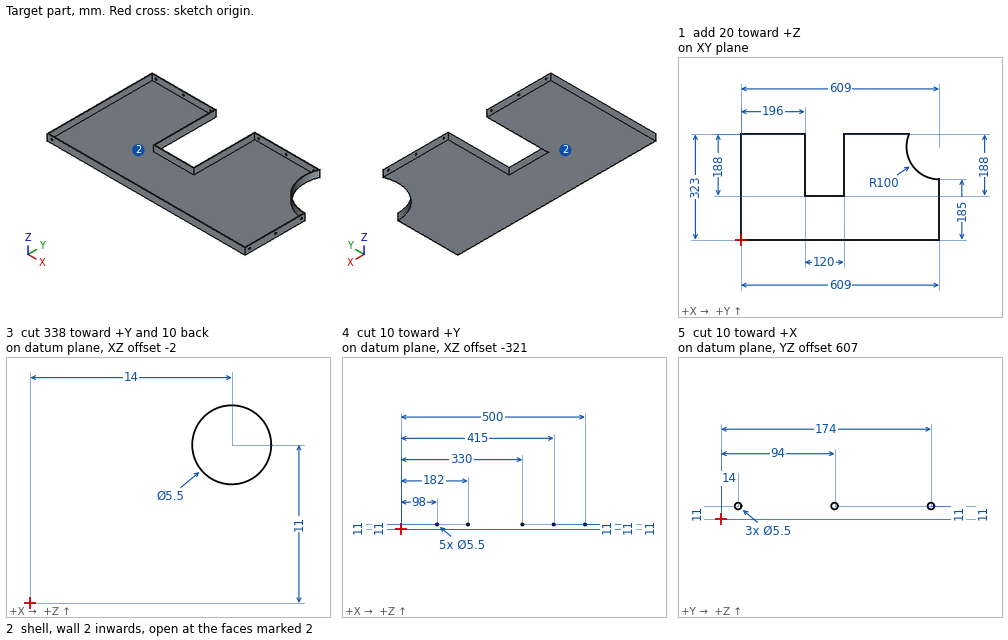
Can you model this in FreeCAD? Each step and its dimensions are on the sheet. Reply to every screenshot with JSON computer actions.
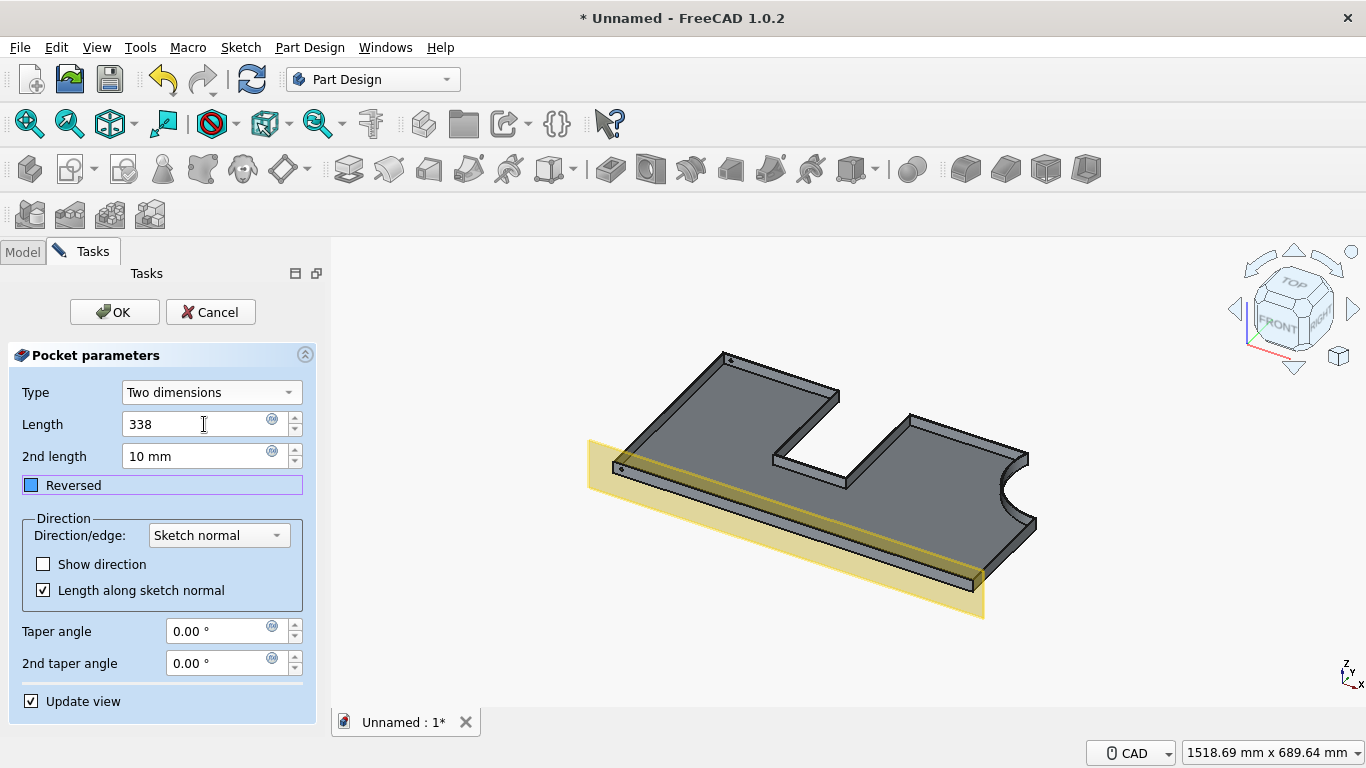
{"action": "left_click", "coordinate": [115, 312]}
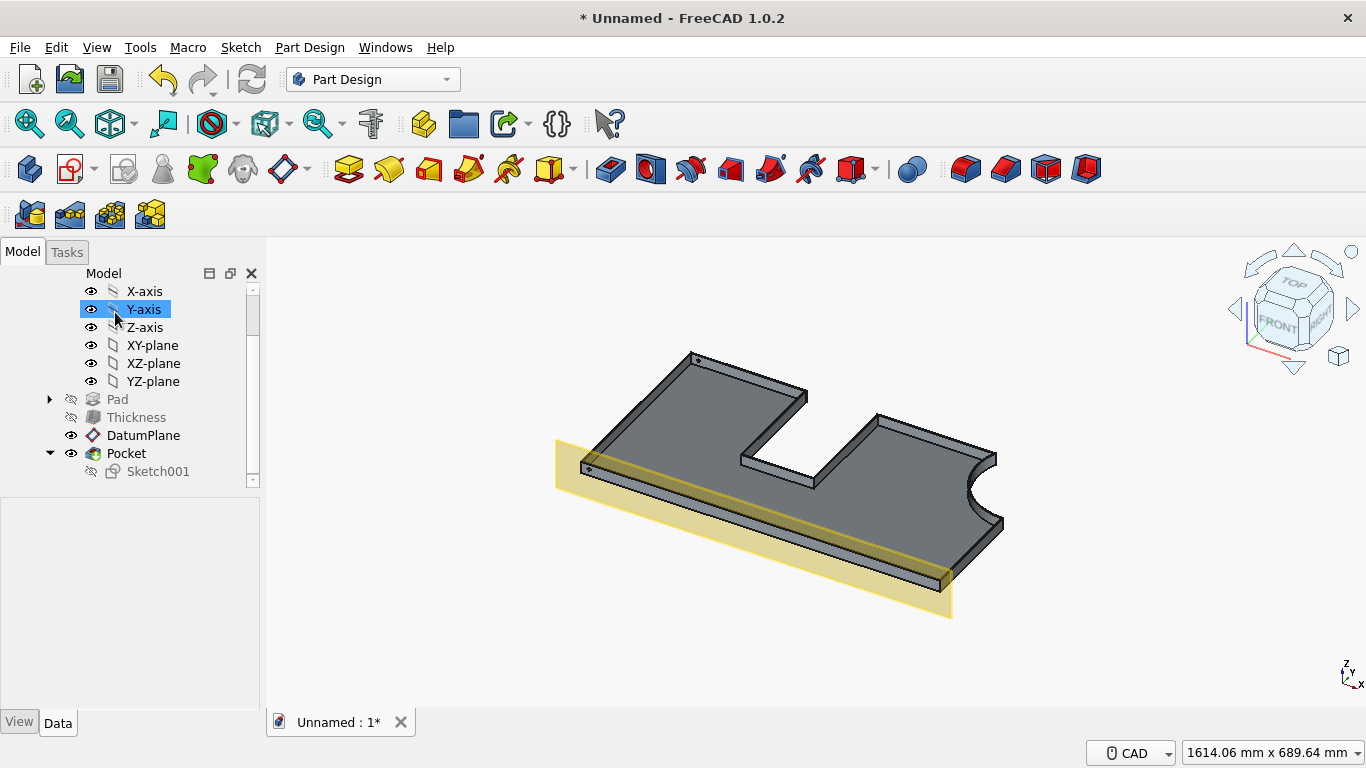
{"action": "left_click", "coordinate": [116, 435]}
{"action": "key", "text": "space"}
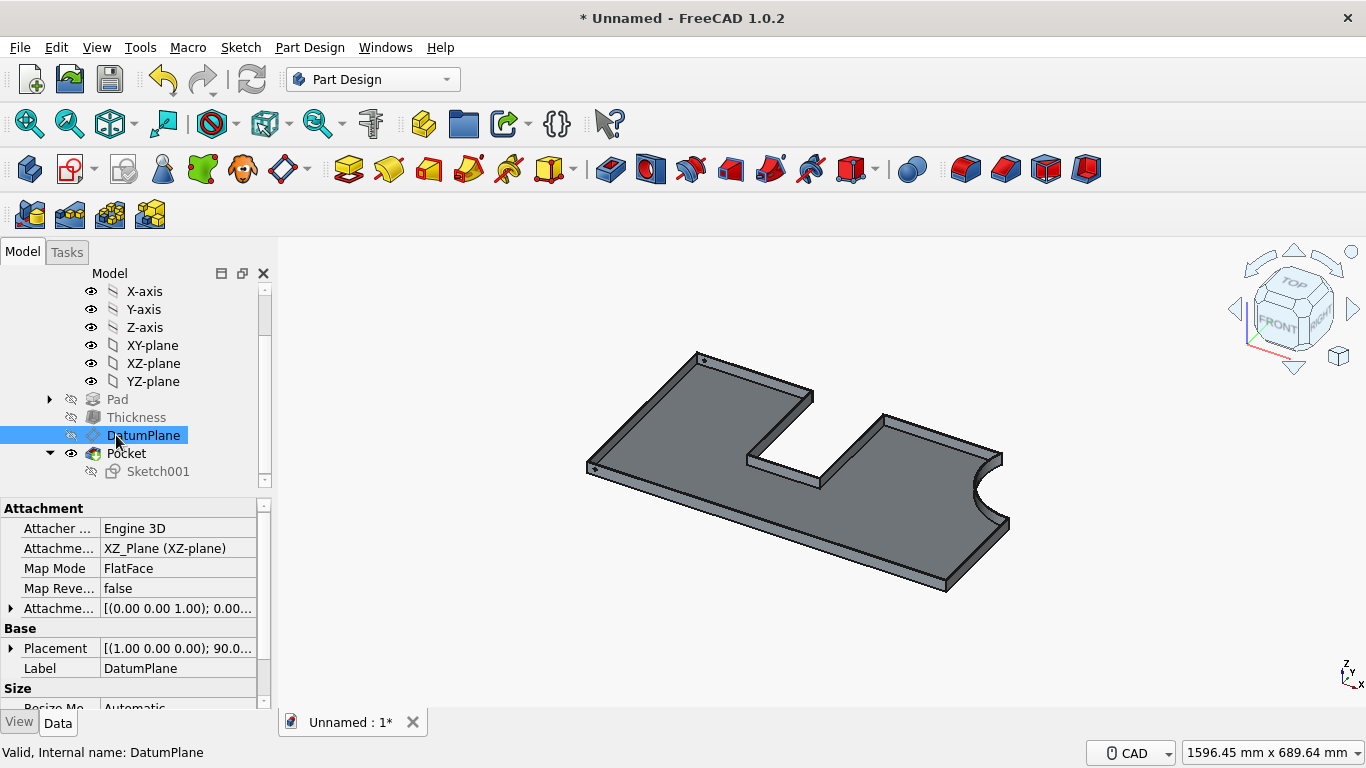
{"action": "scroll", "coordinate": [160, 377], "scroll_direction": "down", "scroll_amount": 3}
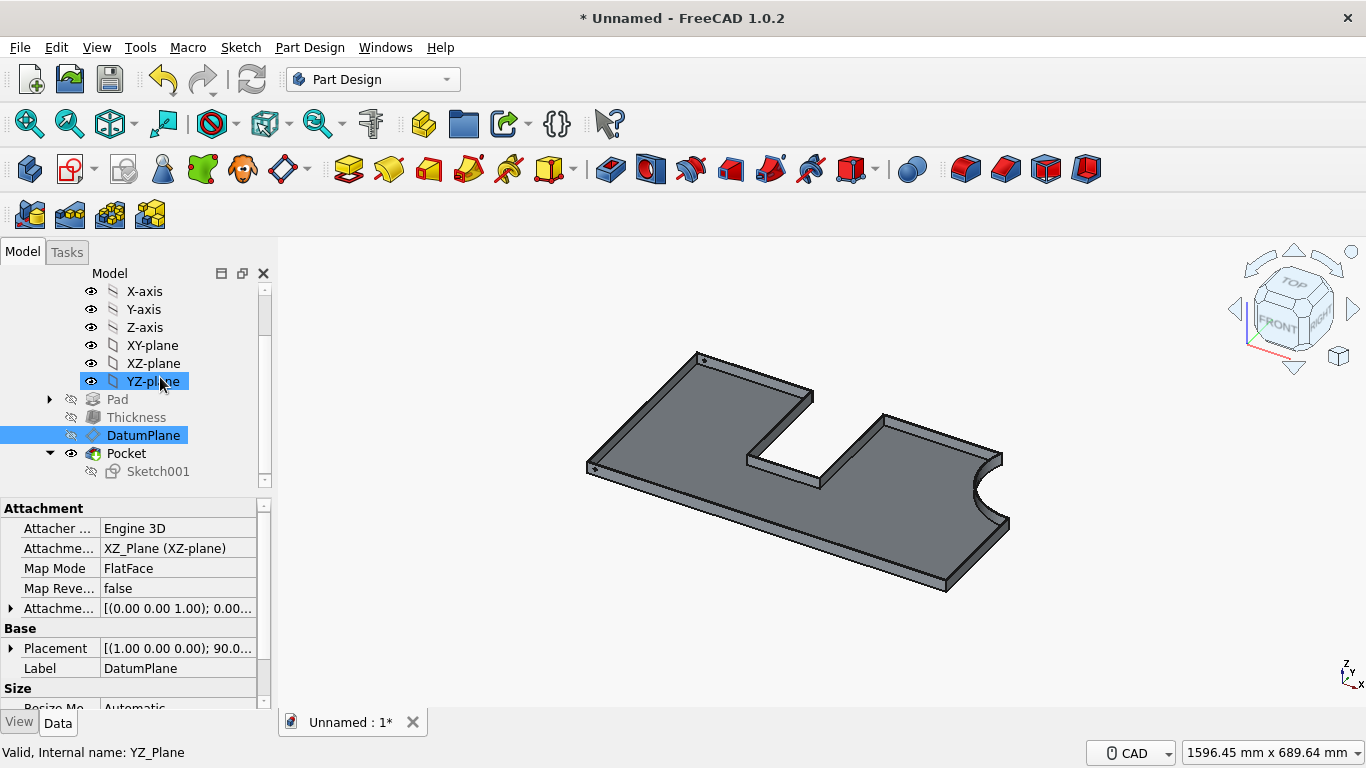
{"action": "scroll", "coordinate": [160, 377], "scroll_direction": "up", "scroll_amount": 15}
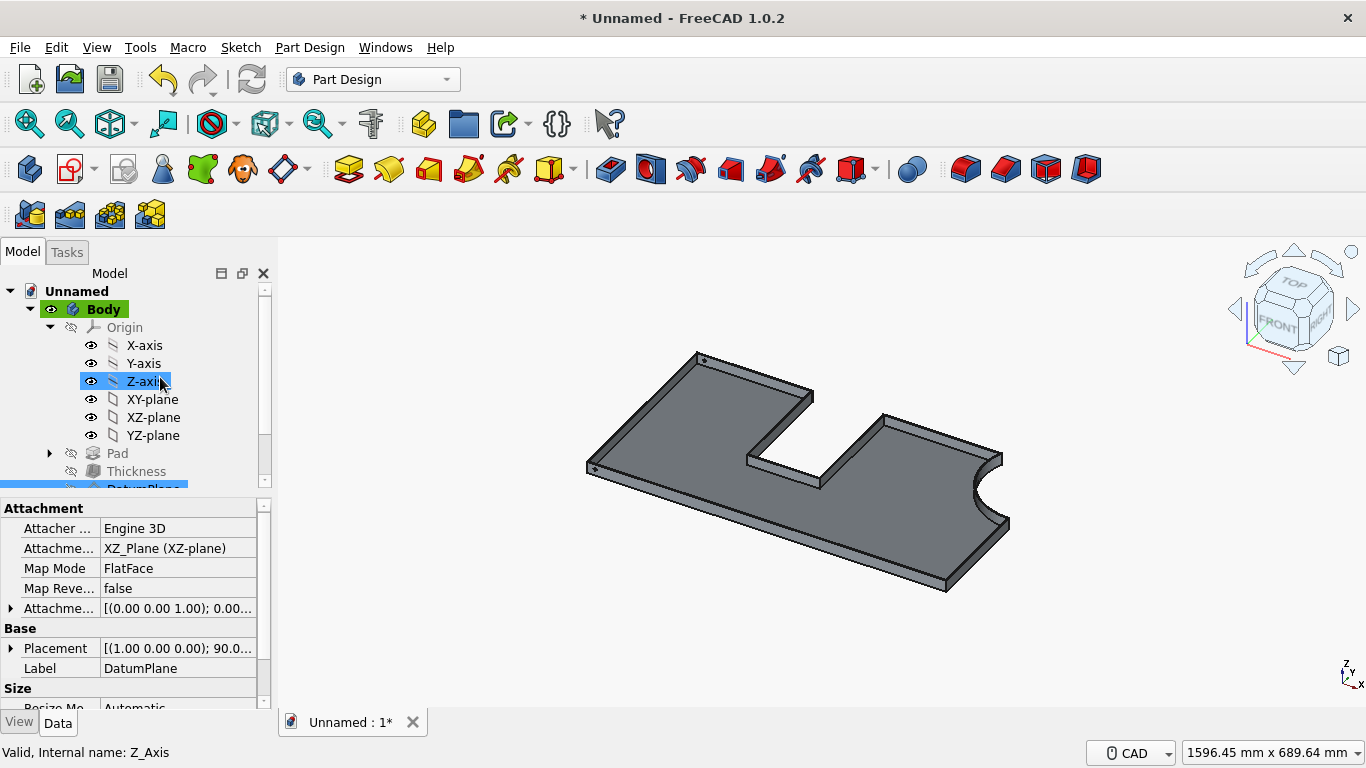
{"action": "left_click", "coordinate": [136, 417]}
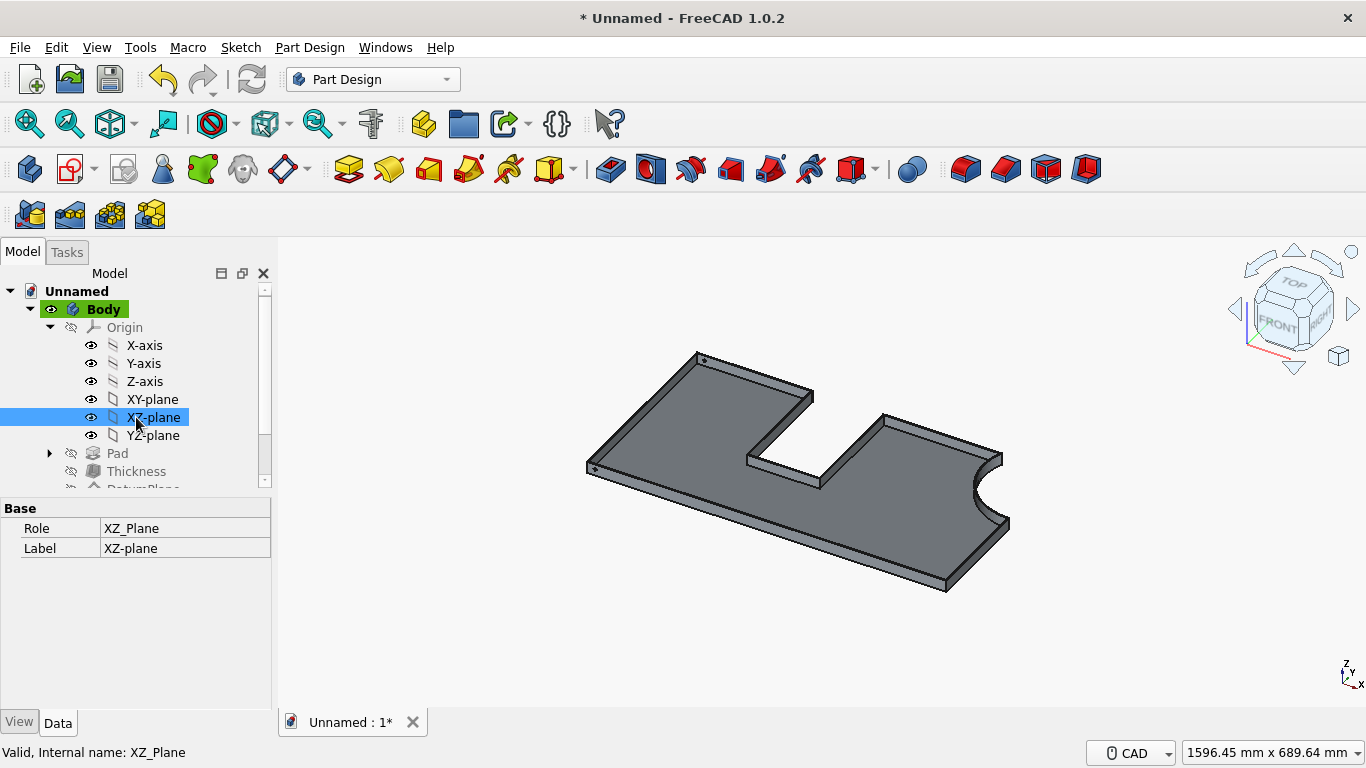
{"action": "left_click", "coordinate": [284, 170]}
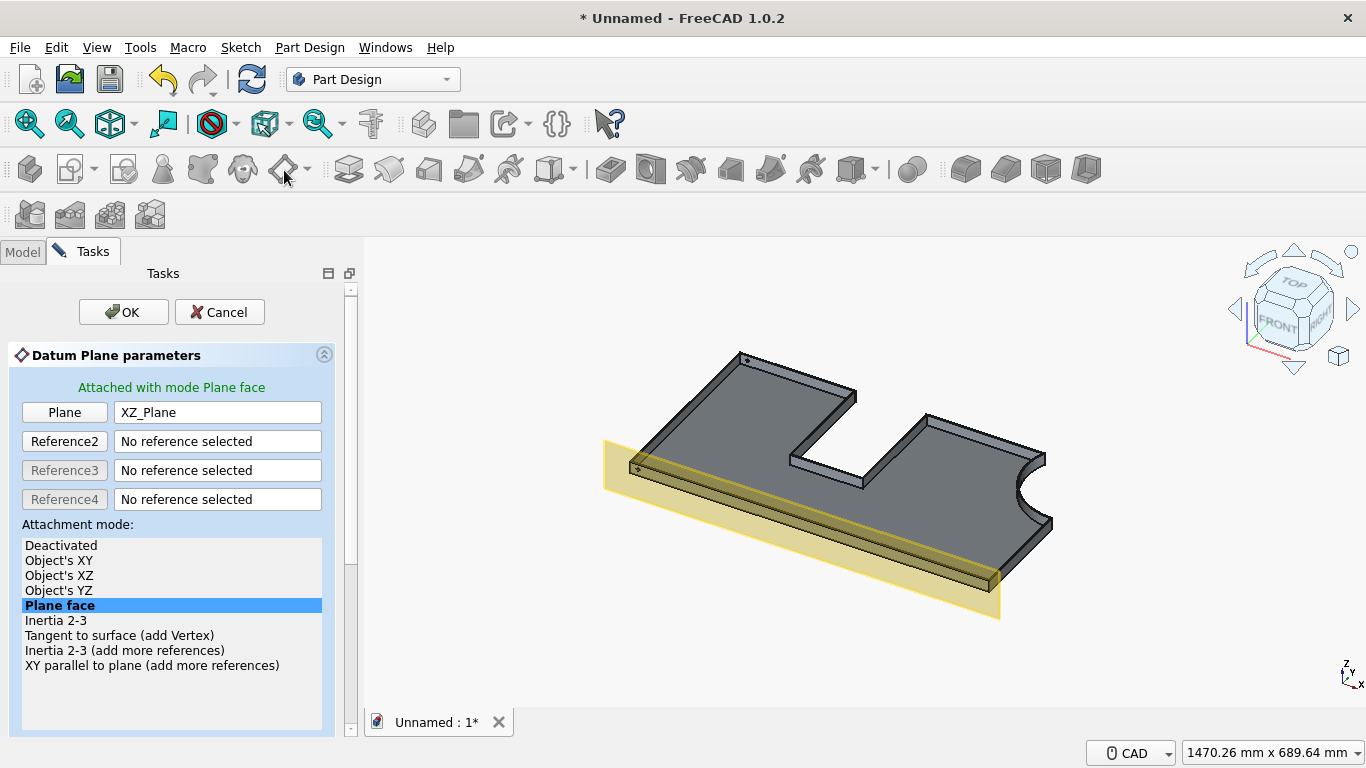
{"action": "scroll", "coordinate": [351, 510], "scroll_direction": "down", "scroll_amount": 3}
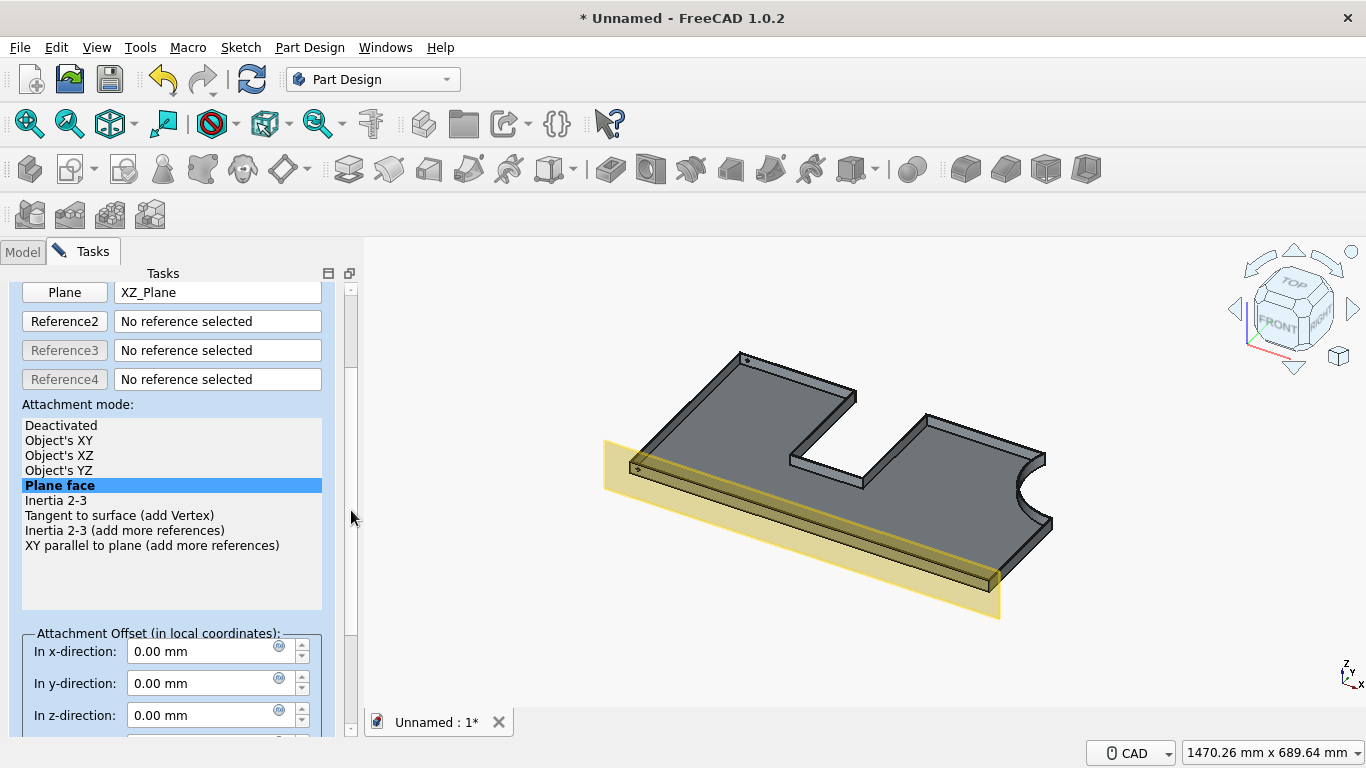
{"action": "triple_click", "coordinate": [210, 655]}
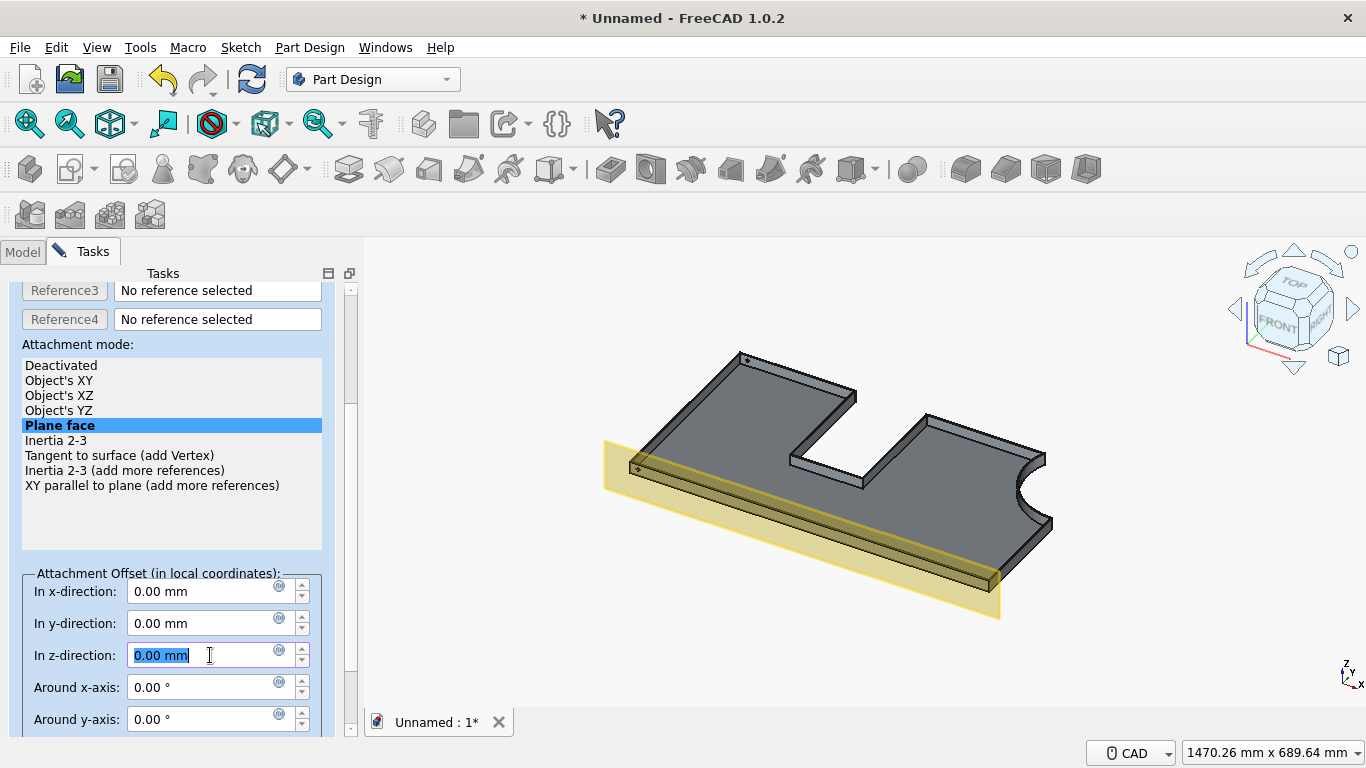
{"action": "type", "text": "-321"}
{"action": "key", "text": "Tab"}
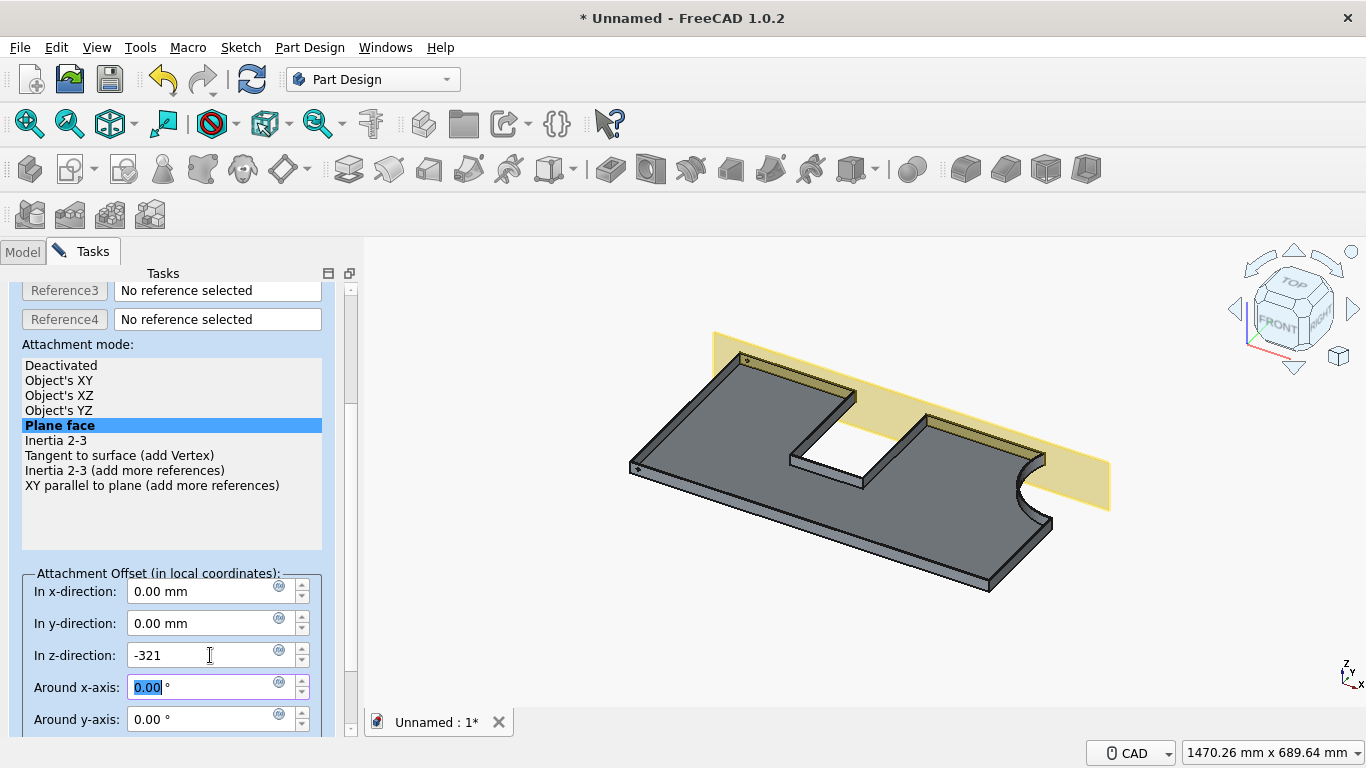
{"action": "scroll", "coordinate": [351, 510], "scroll_direction": "up", "scroll_amount": 4}